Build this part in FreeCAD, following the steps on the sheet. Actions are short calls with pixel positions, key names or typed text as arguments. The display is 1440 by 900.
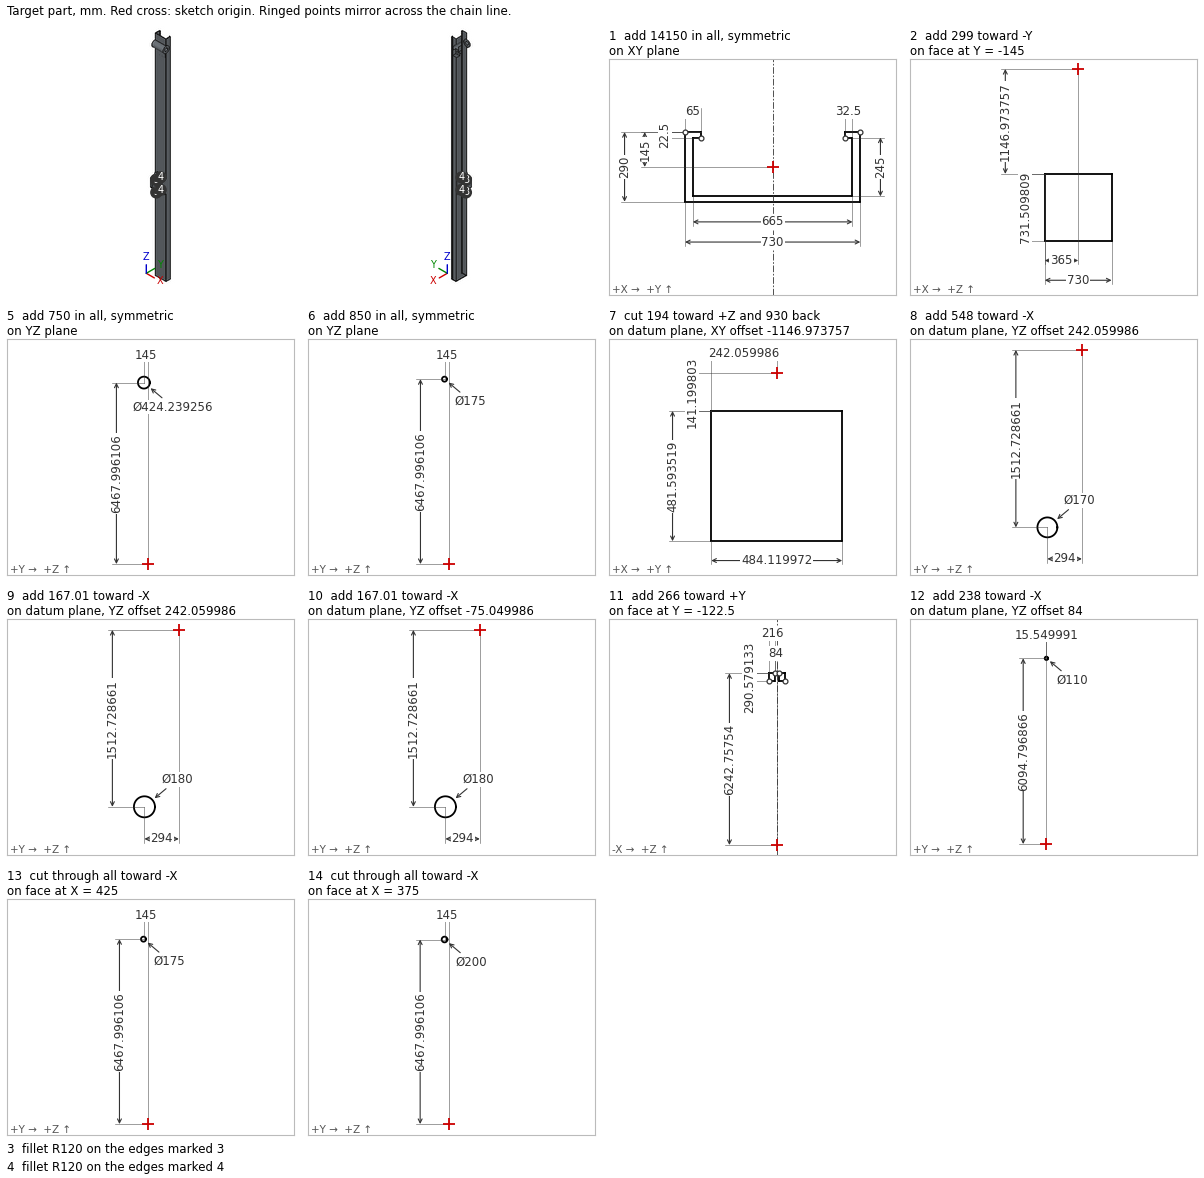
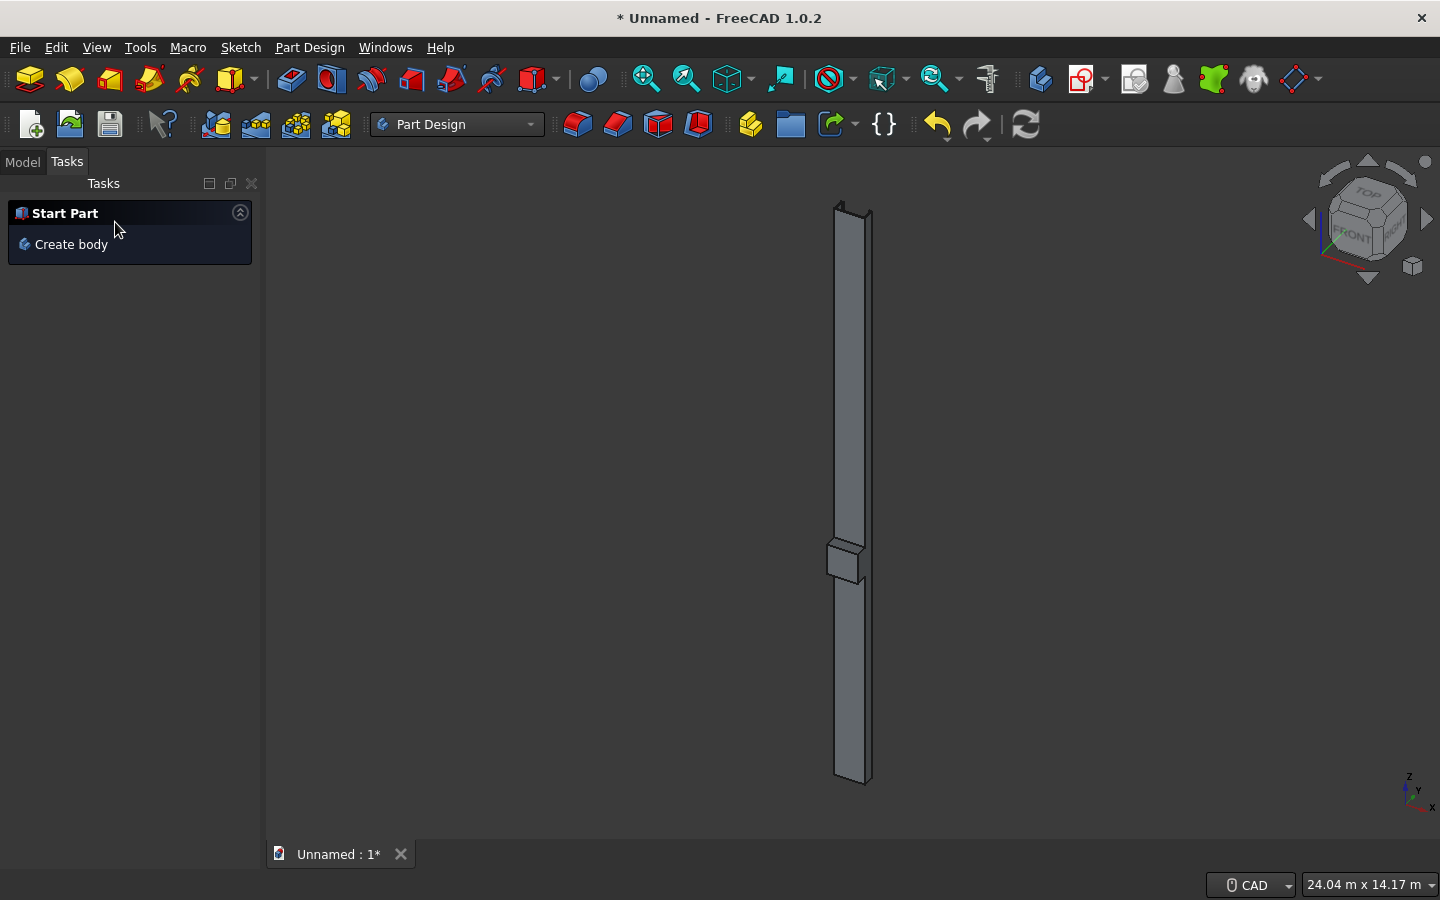
click(842, 549)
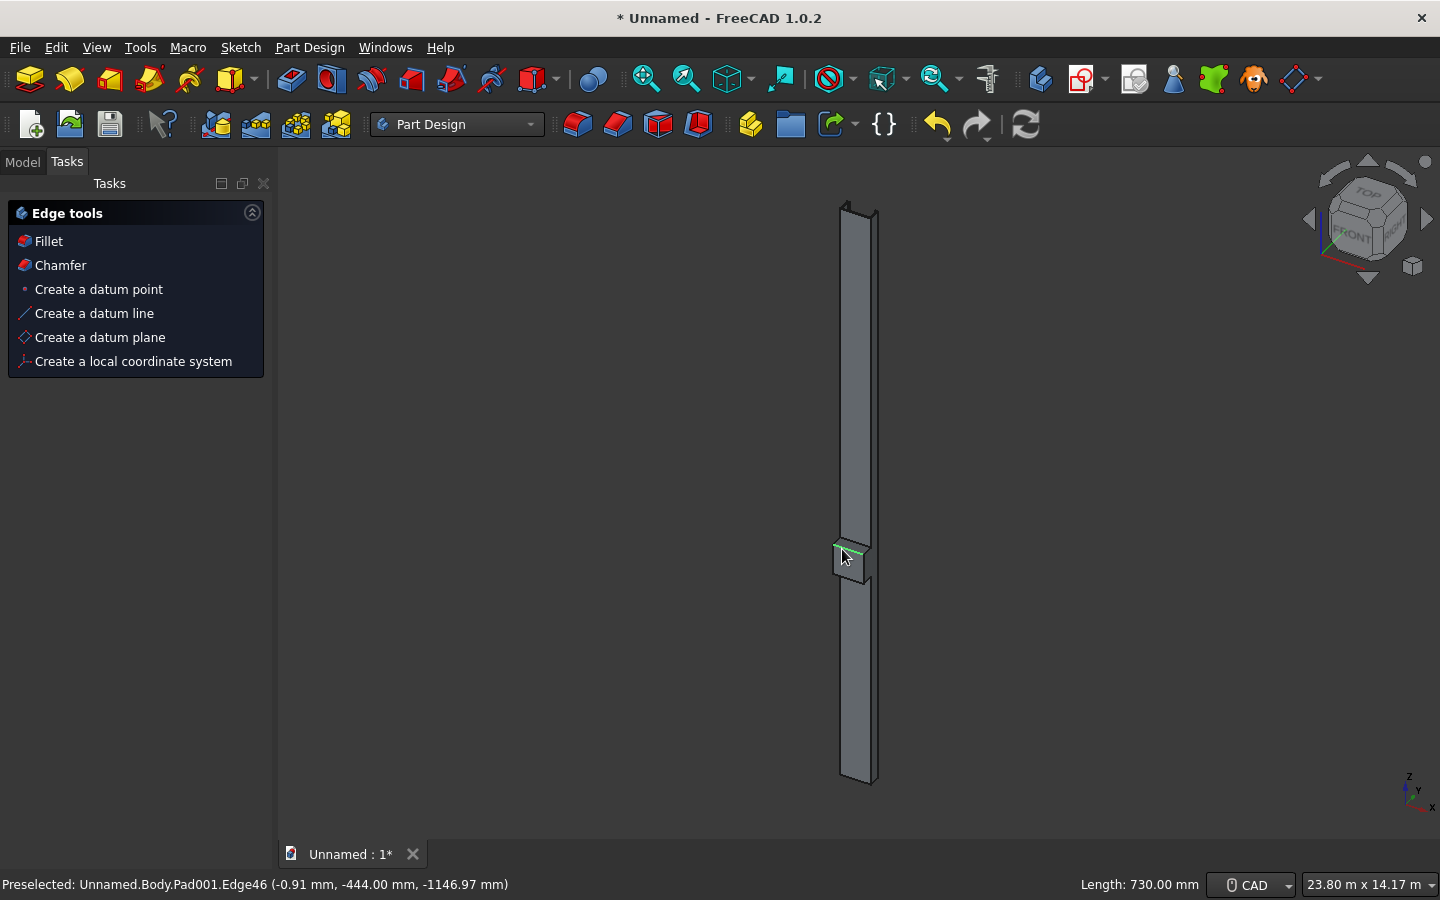
key(0)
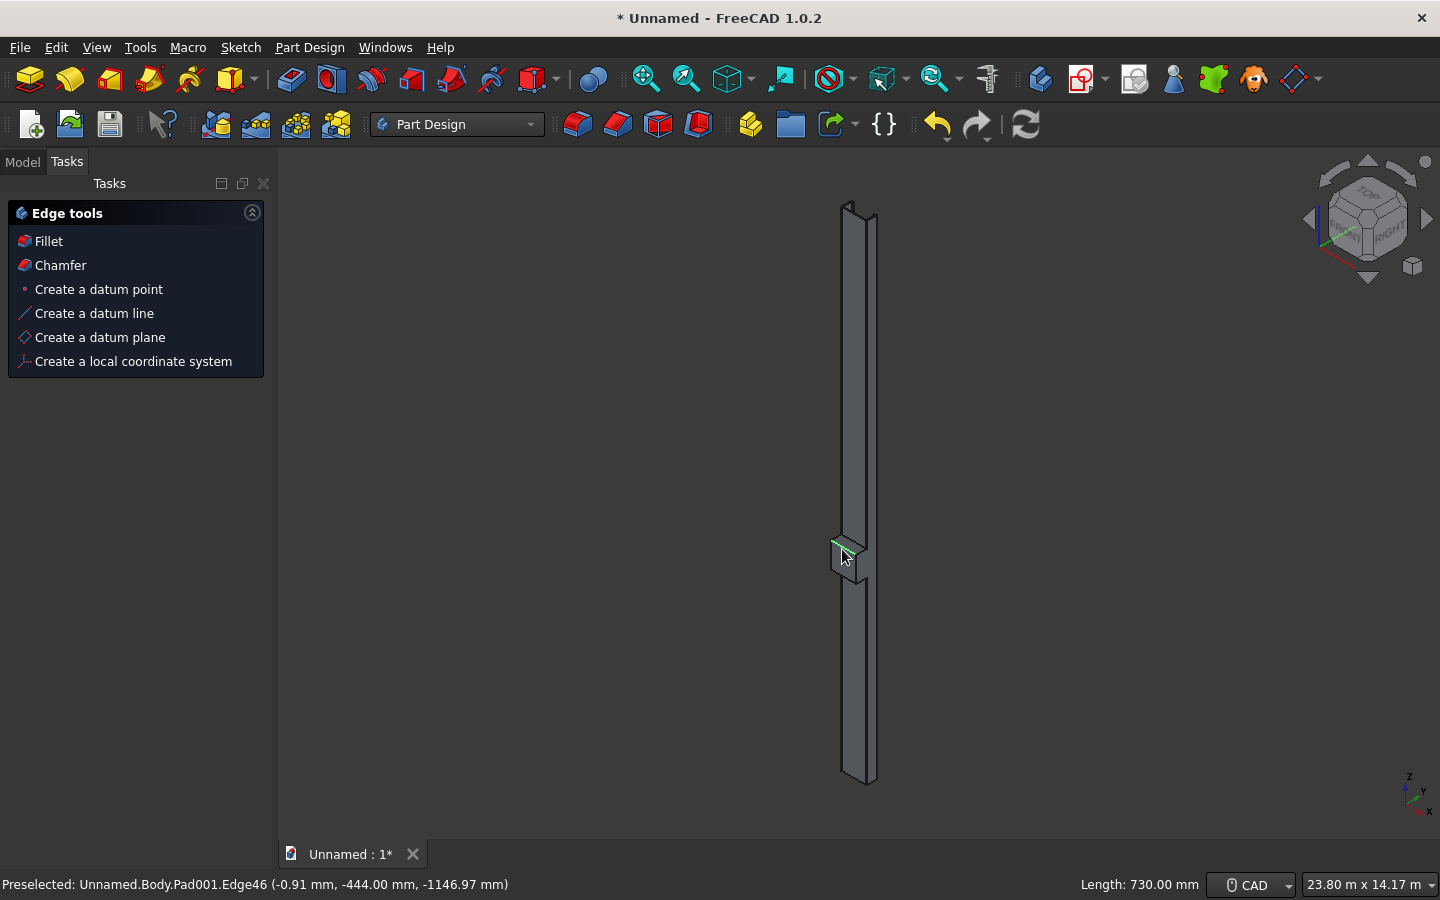
key(2)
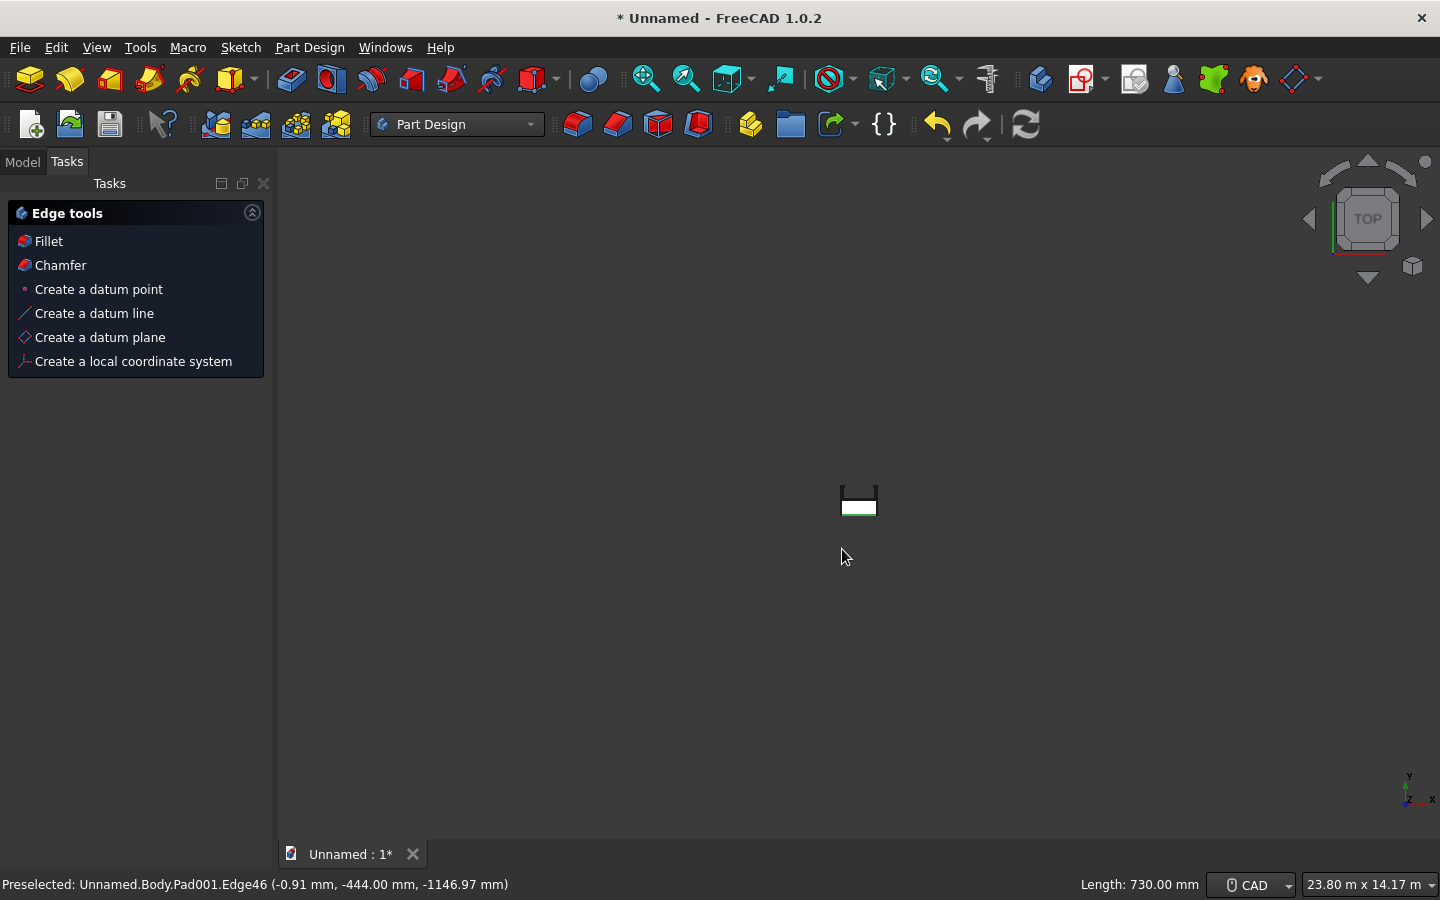
click(648, 80)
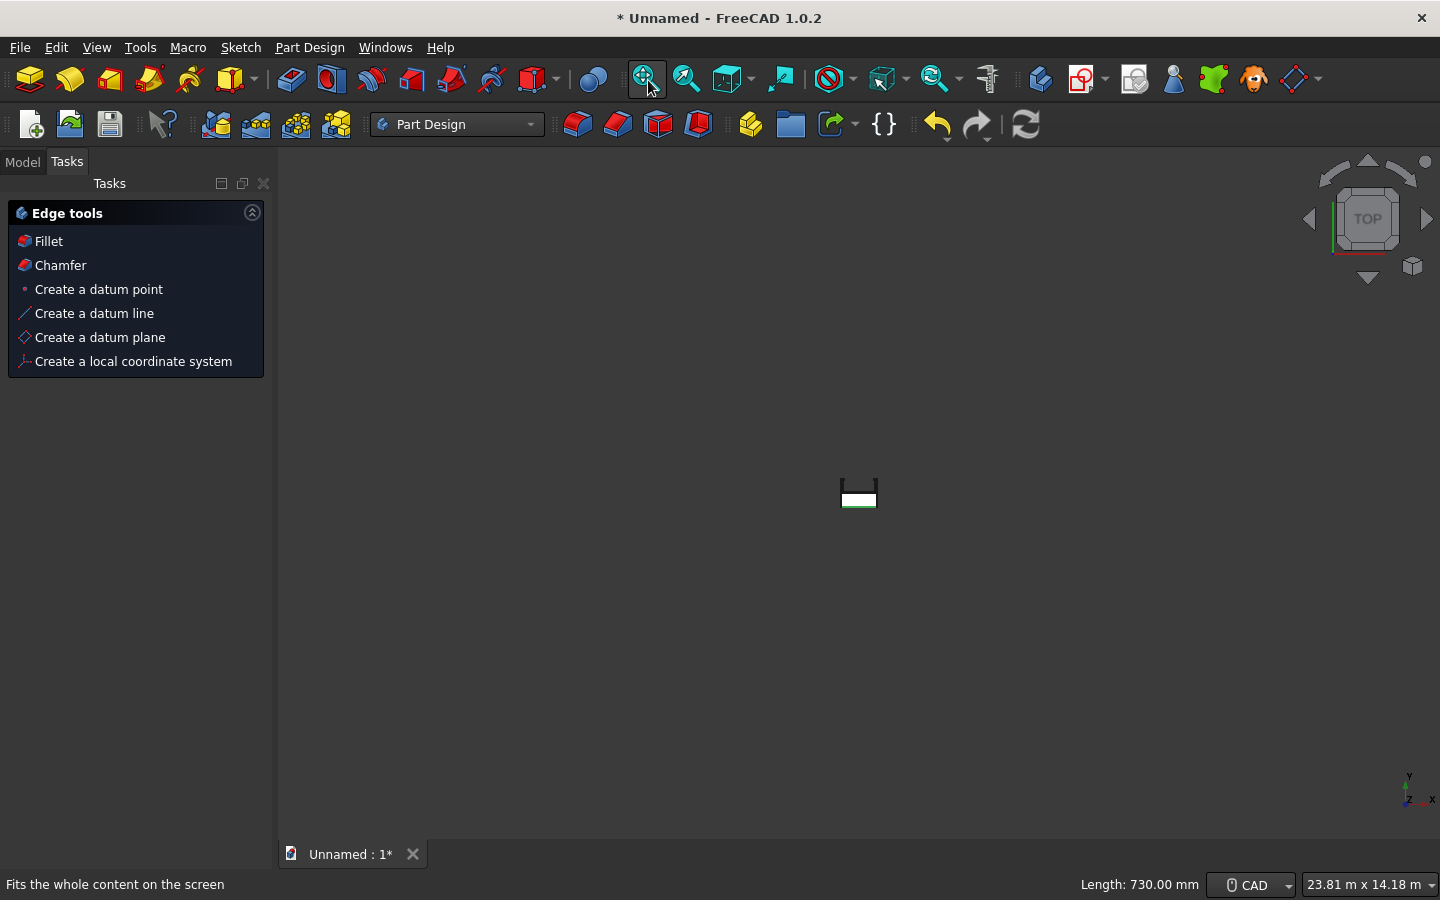
key(1)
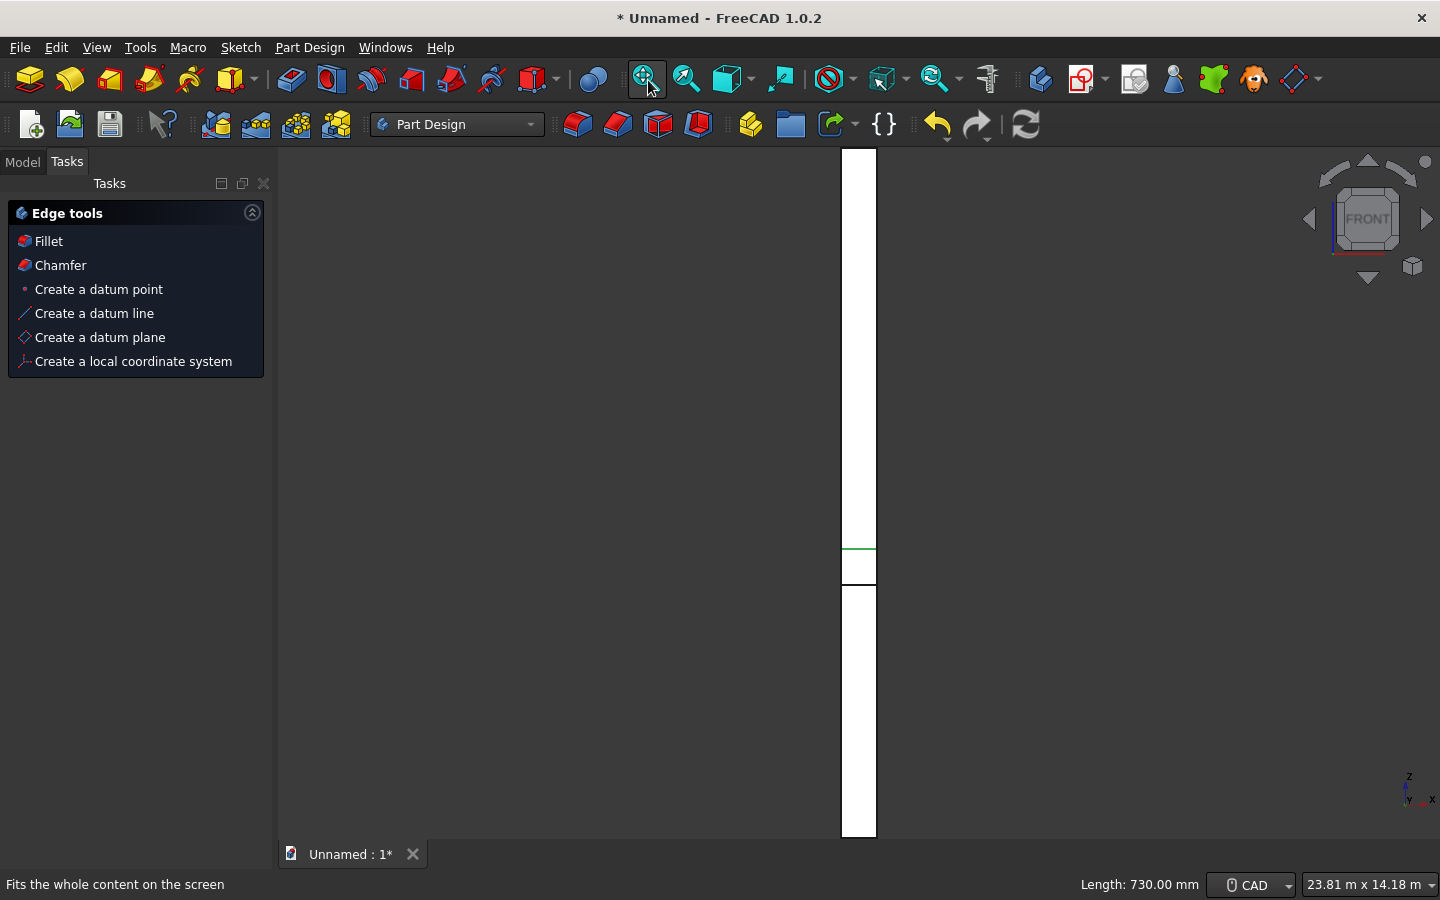
click(859, 584, ctrl)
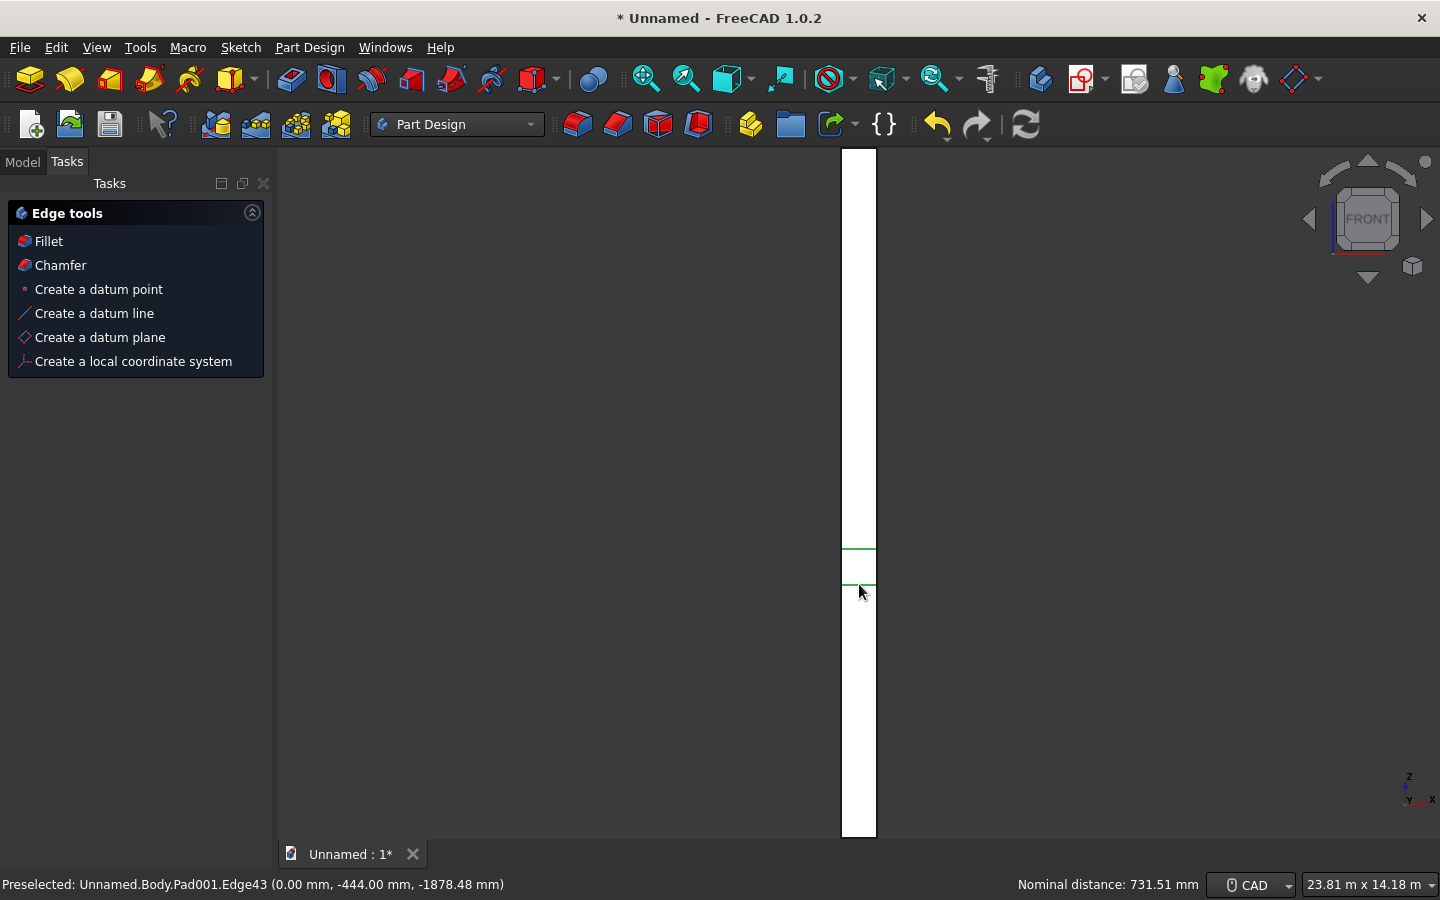
click(578, 124)